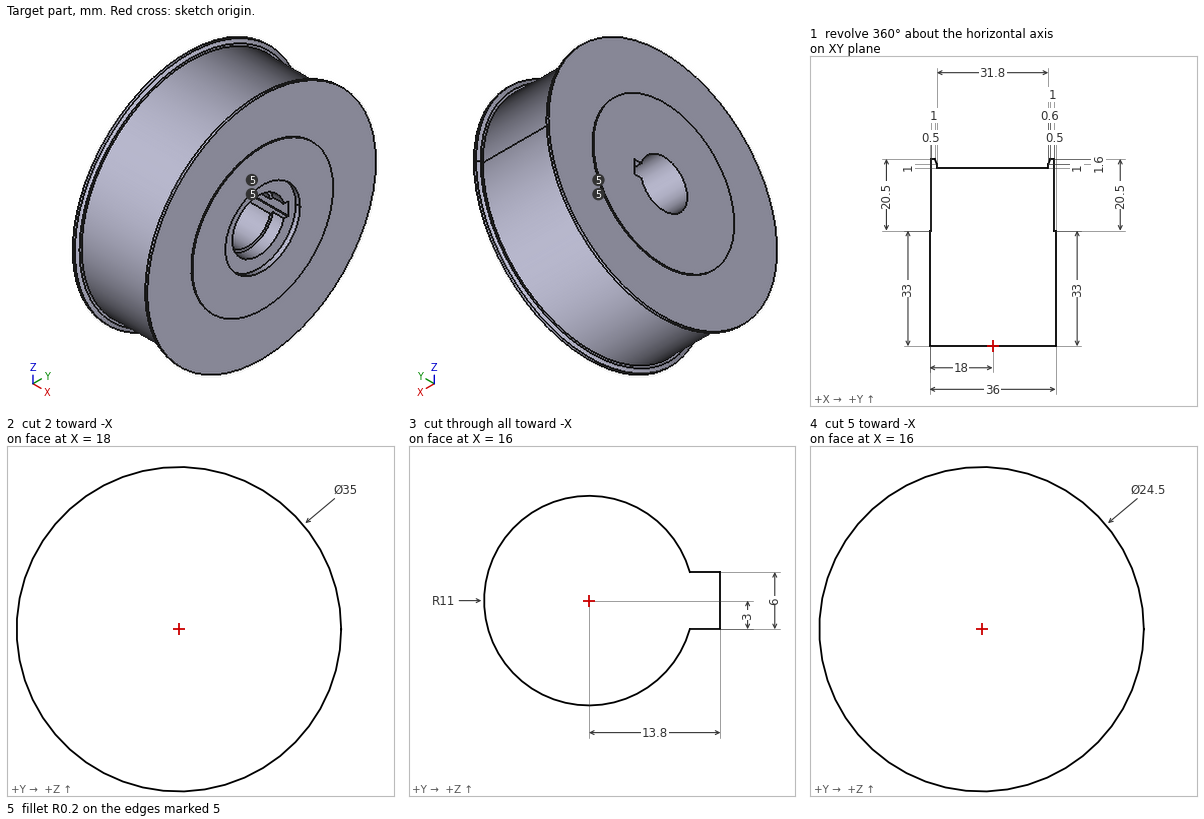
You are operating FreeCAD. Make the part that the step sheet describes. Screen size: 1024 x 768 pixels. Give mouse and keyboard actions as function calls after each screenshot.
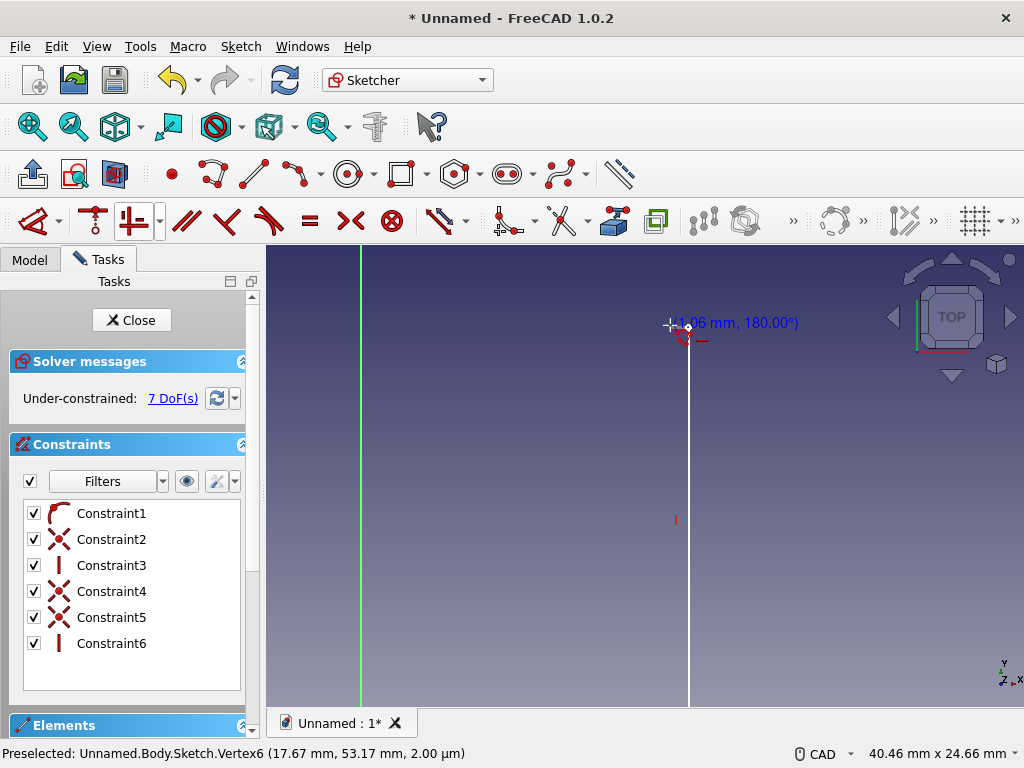
click(670, 325)
click(659, 355)
click(659, 374)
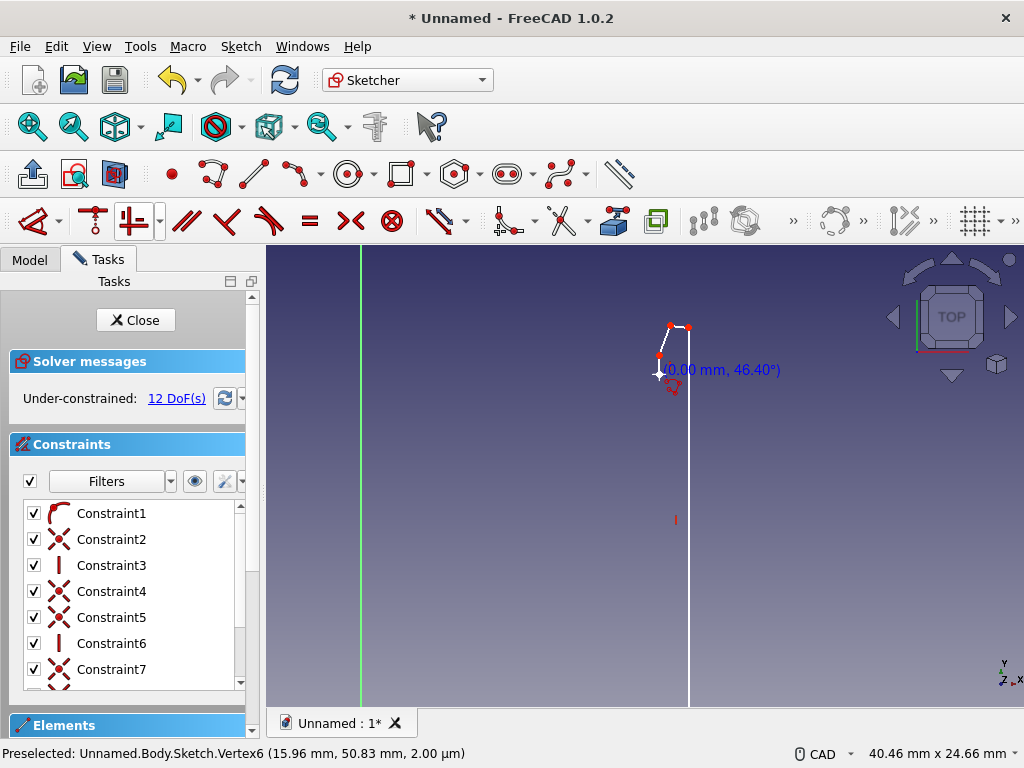
scroll(669, 325, down, 6)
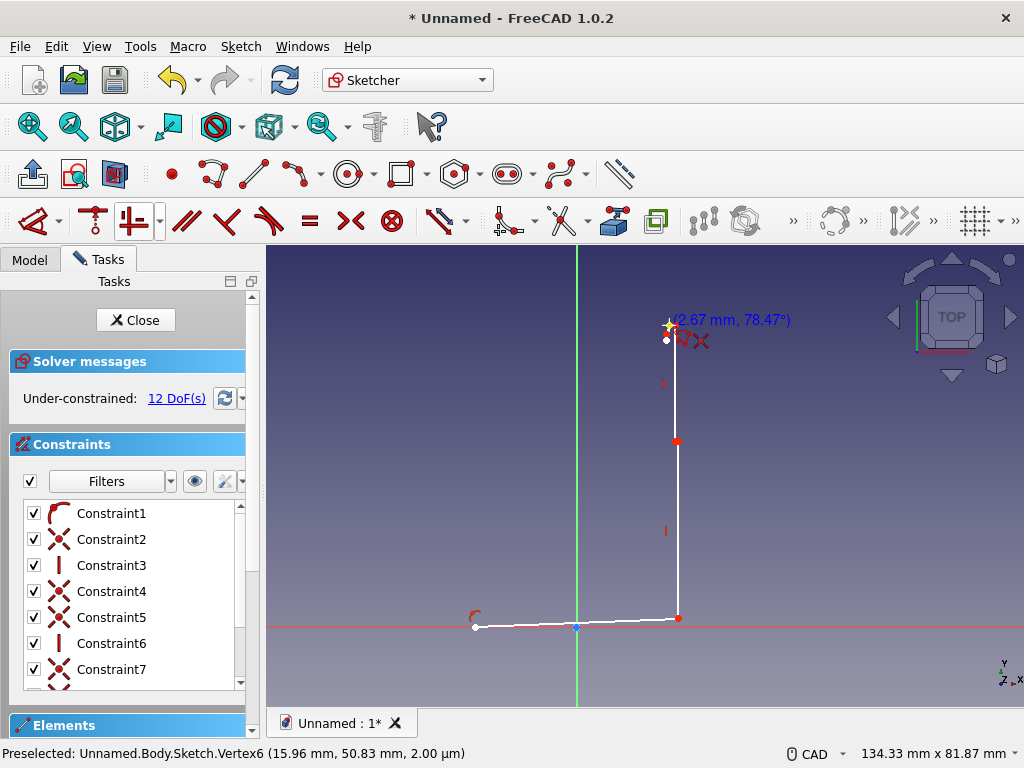
click(487, 340)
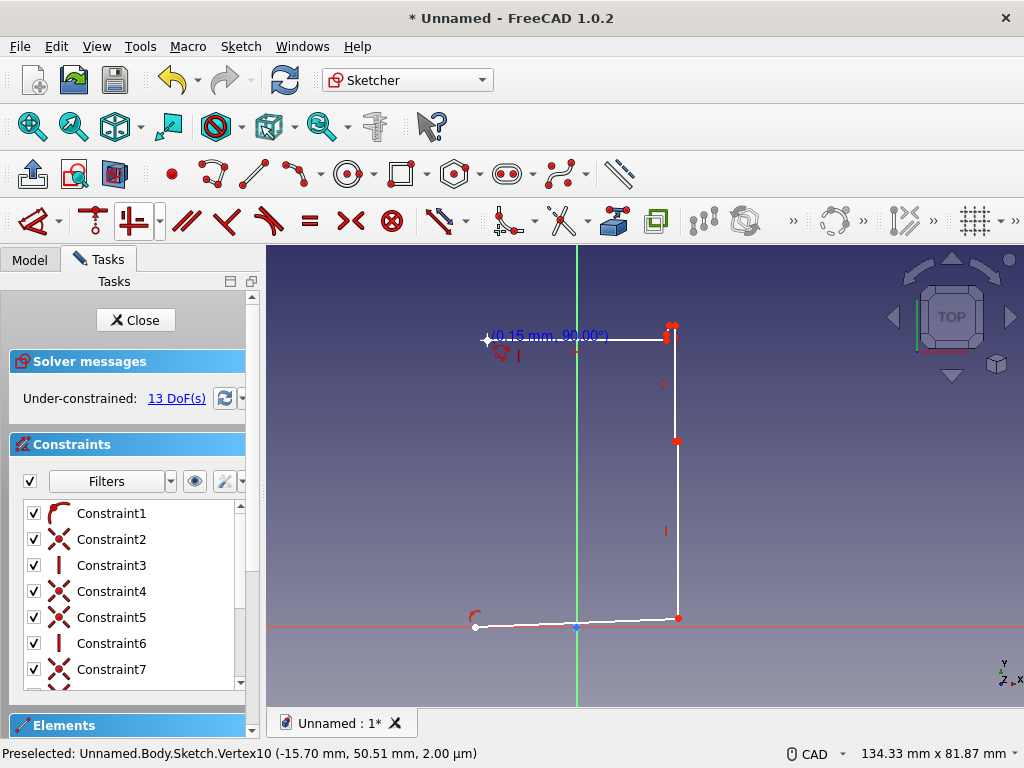
scroll(487, 334, up, 6)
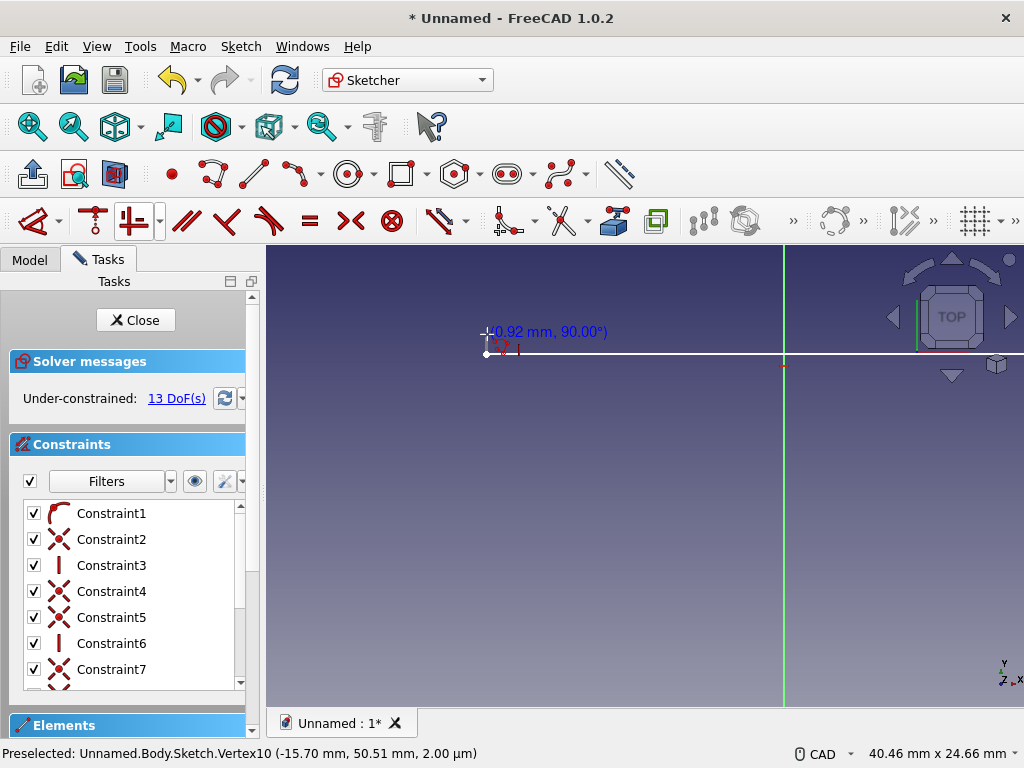
click(486, 334)
click(475, 304)
click(456, 304)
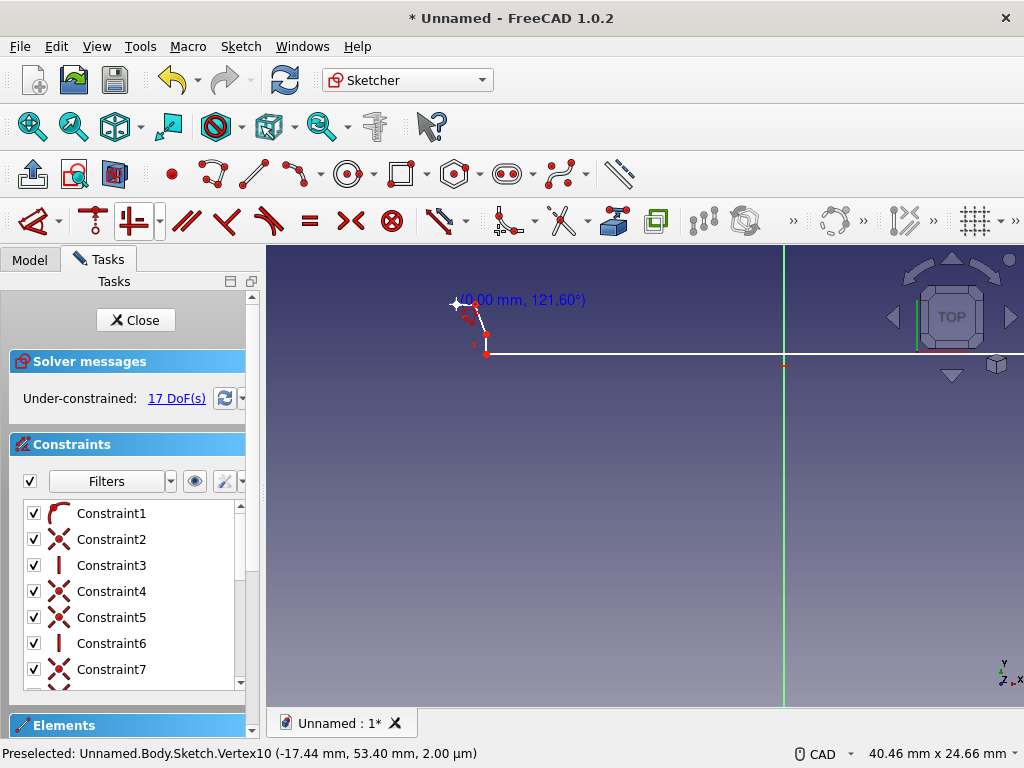
scroll(487, 334, down, 6)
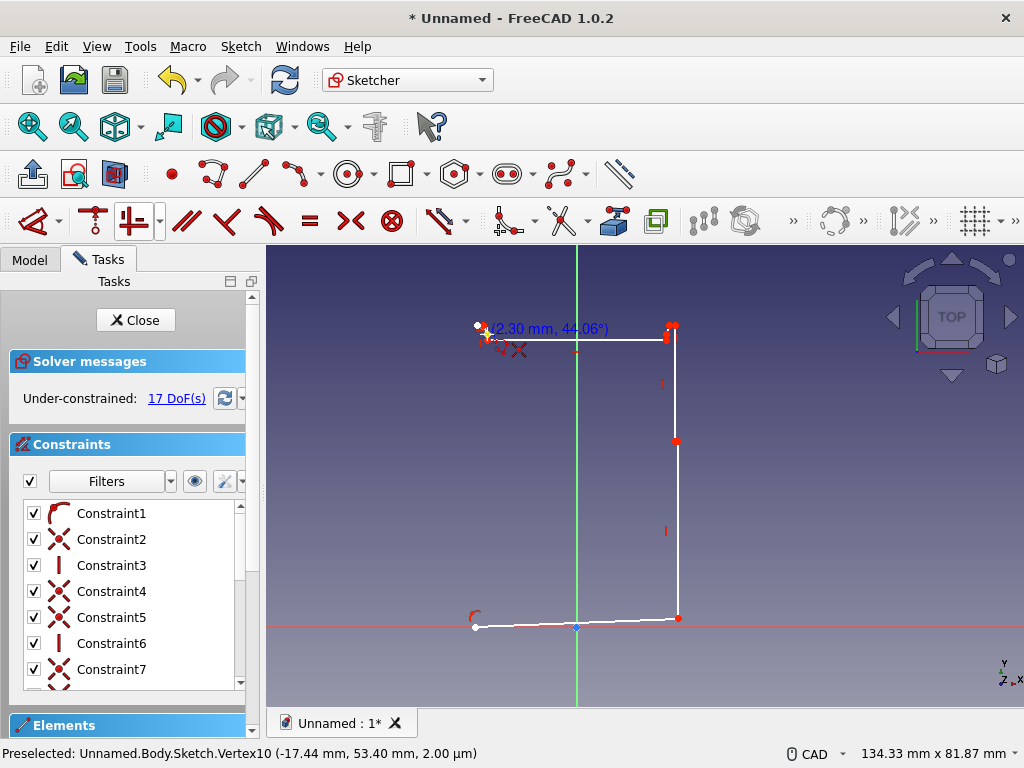
click(478, 441)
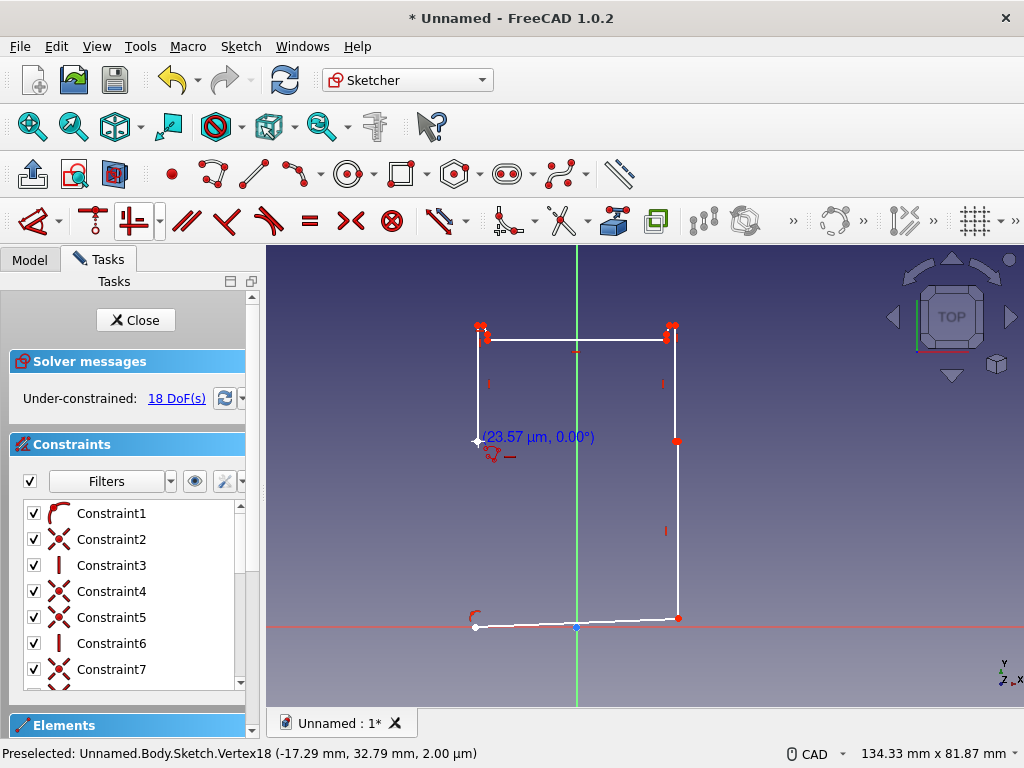
scroll(475, 441, up, 9)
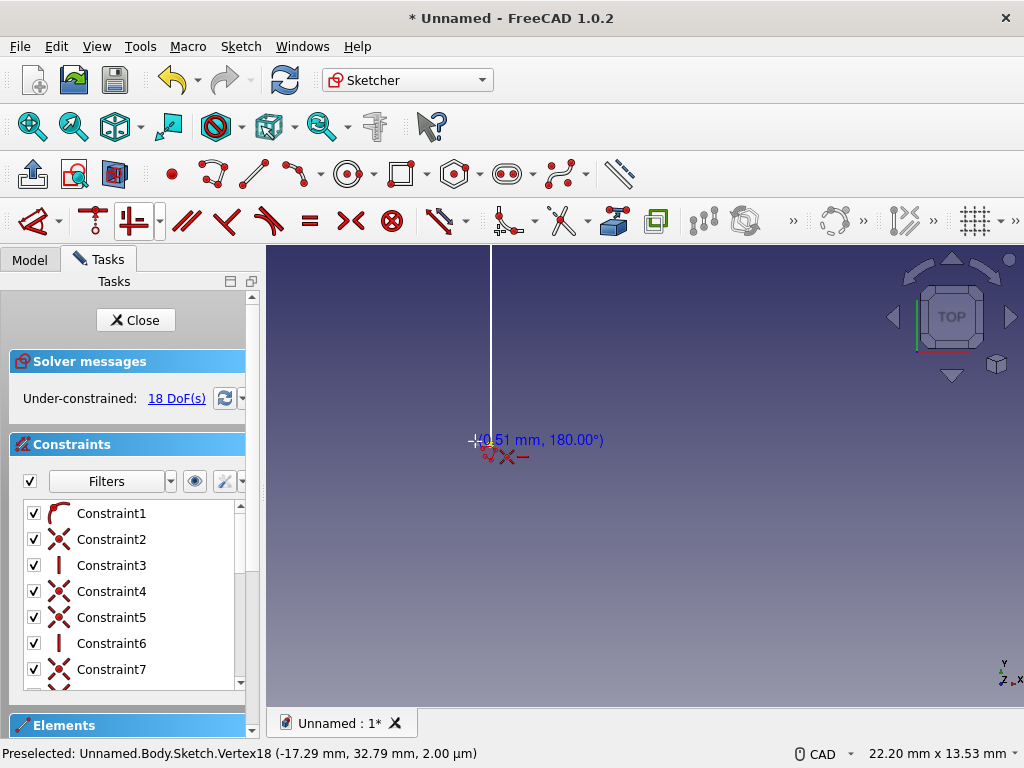
click(474, 439)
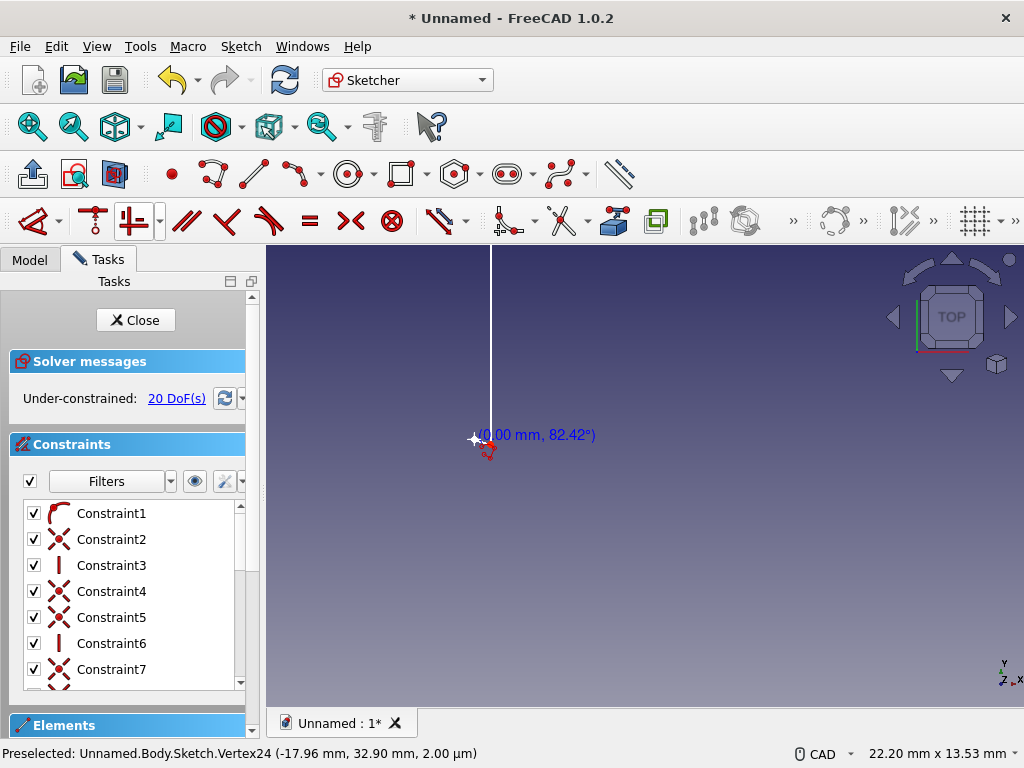
scroll(475, 441, down, 9)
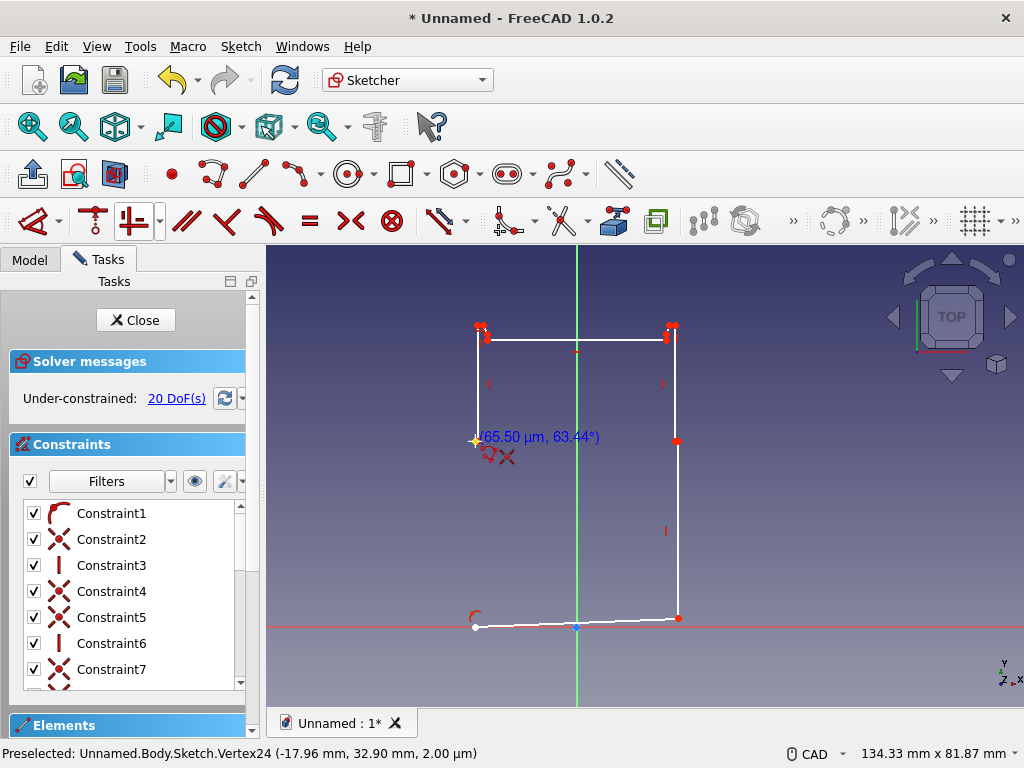
click(475, 627)
key(Escape)
key(Escape)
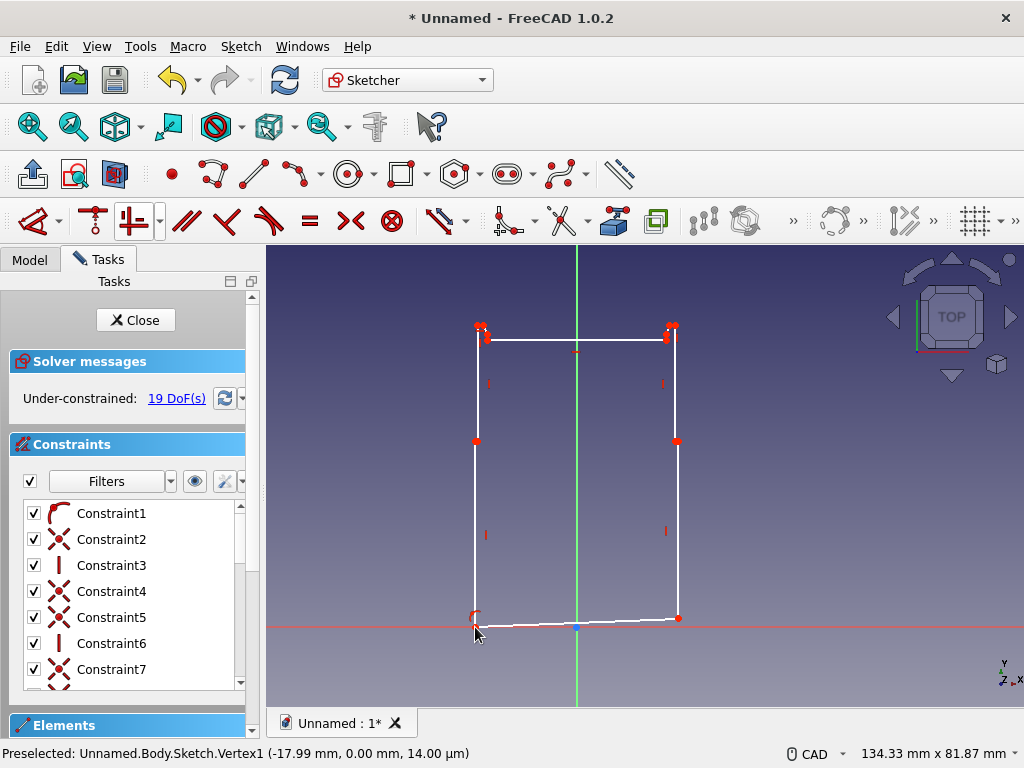
click(536, 625)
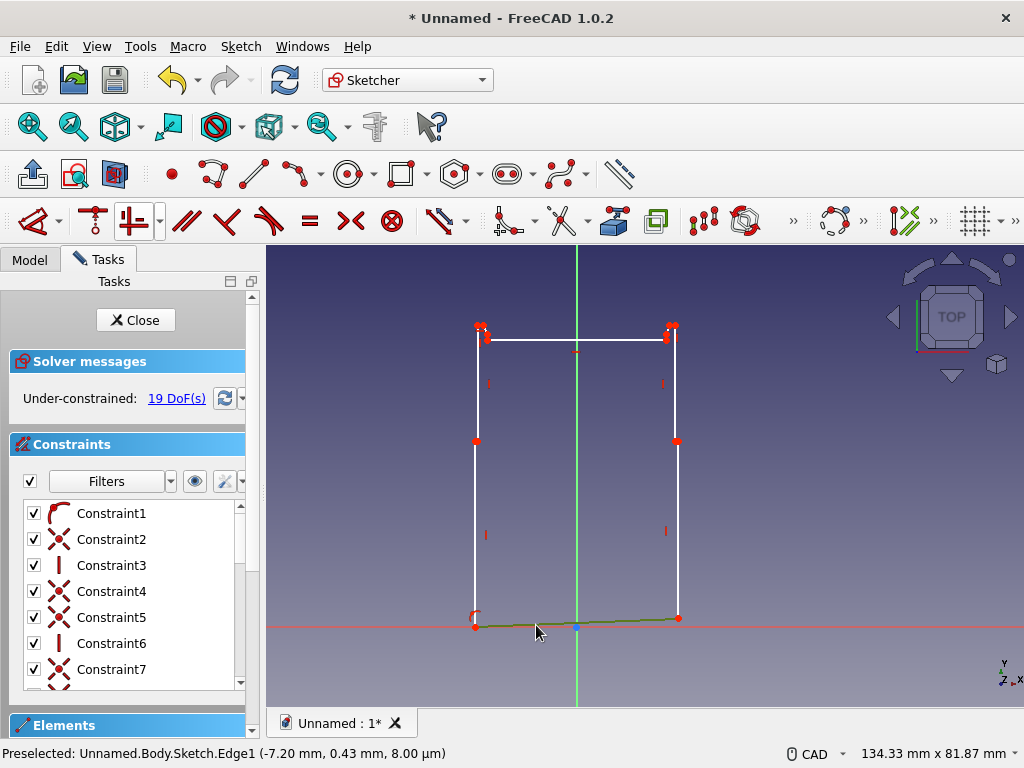
key(h)